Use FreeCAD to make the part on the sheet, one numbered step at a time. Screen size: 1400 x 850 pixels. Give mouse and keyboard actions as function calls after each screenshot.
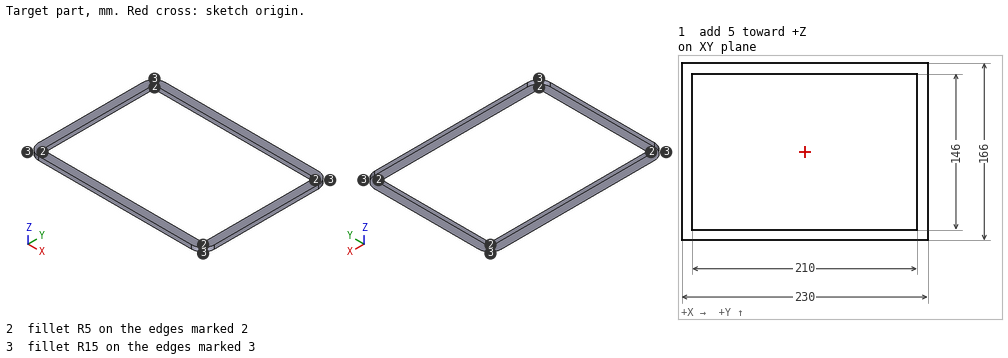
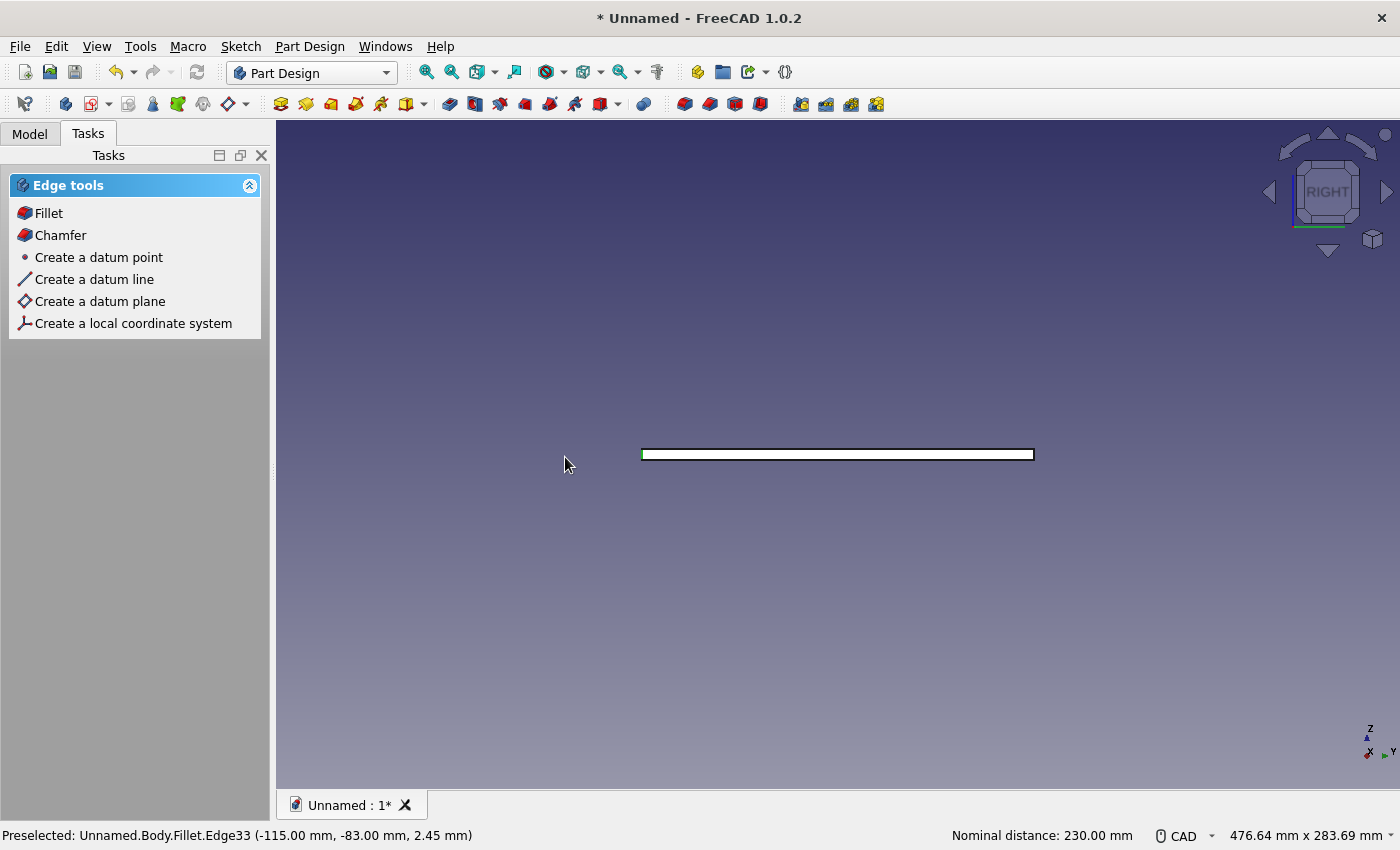
scroll(1034, 453, up, 7)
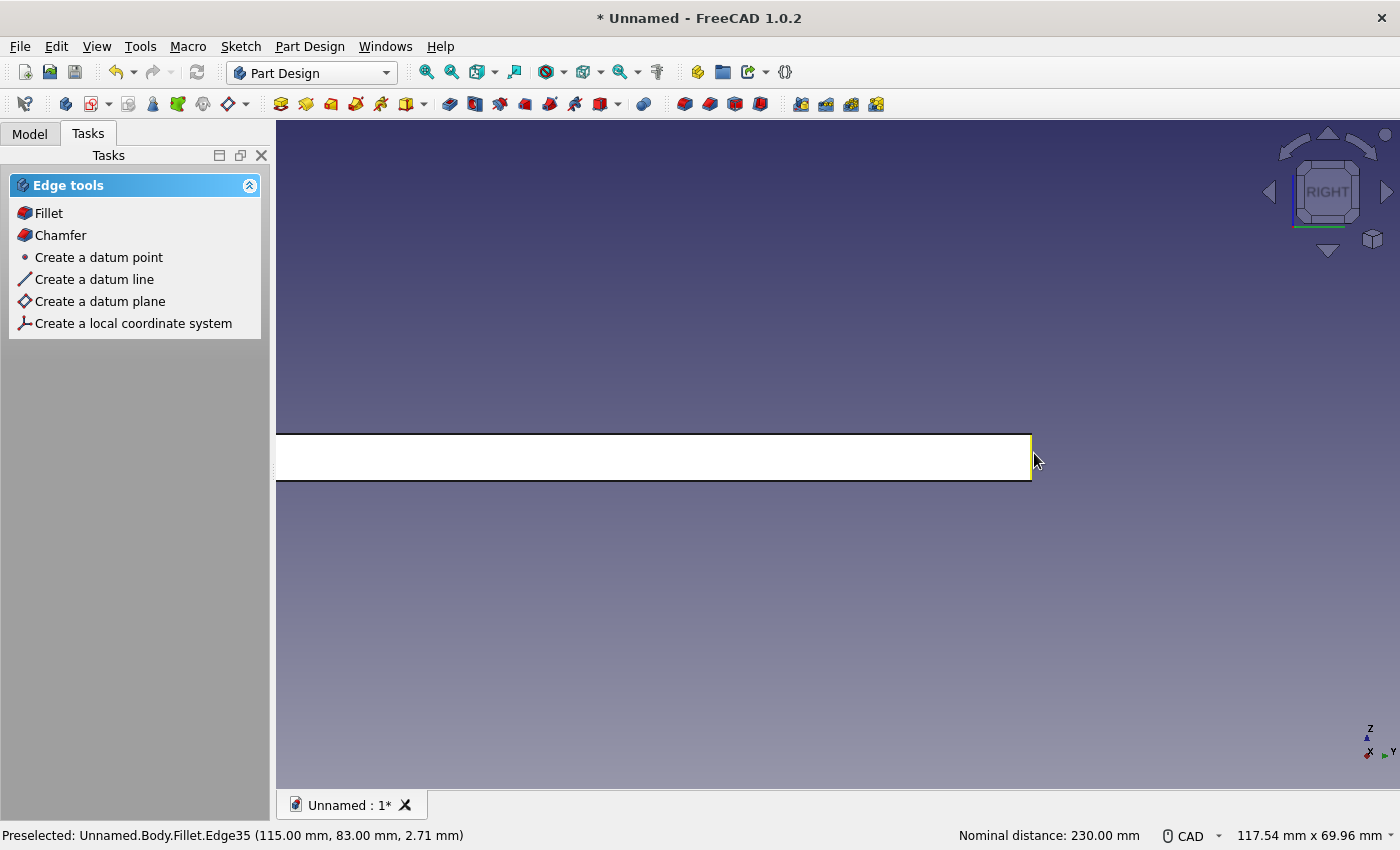
click(1031, 457, ctrl)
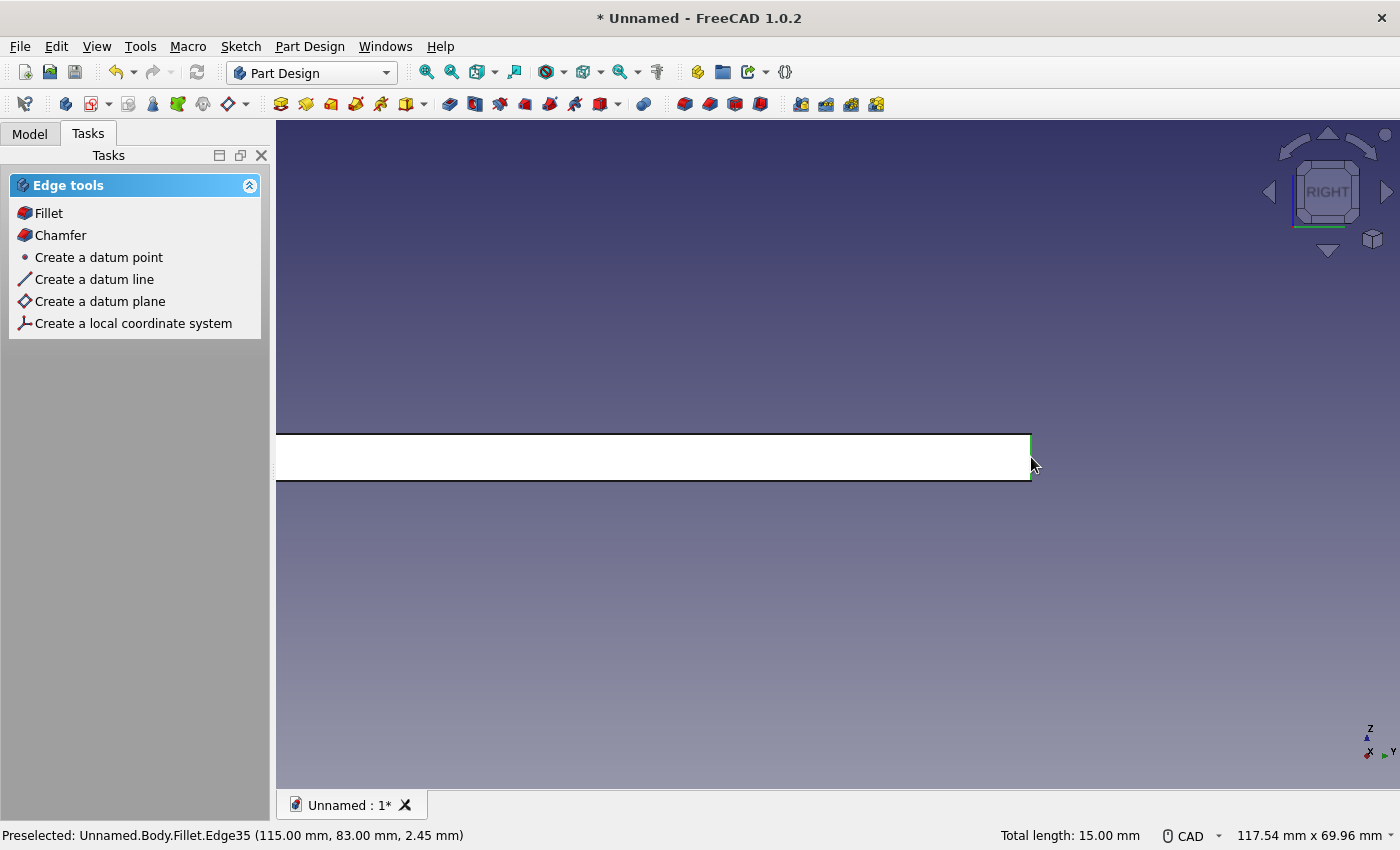
key(v)
key(f)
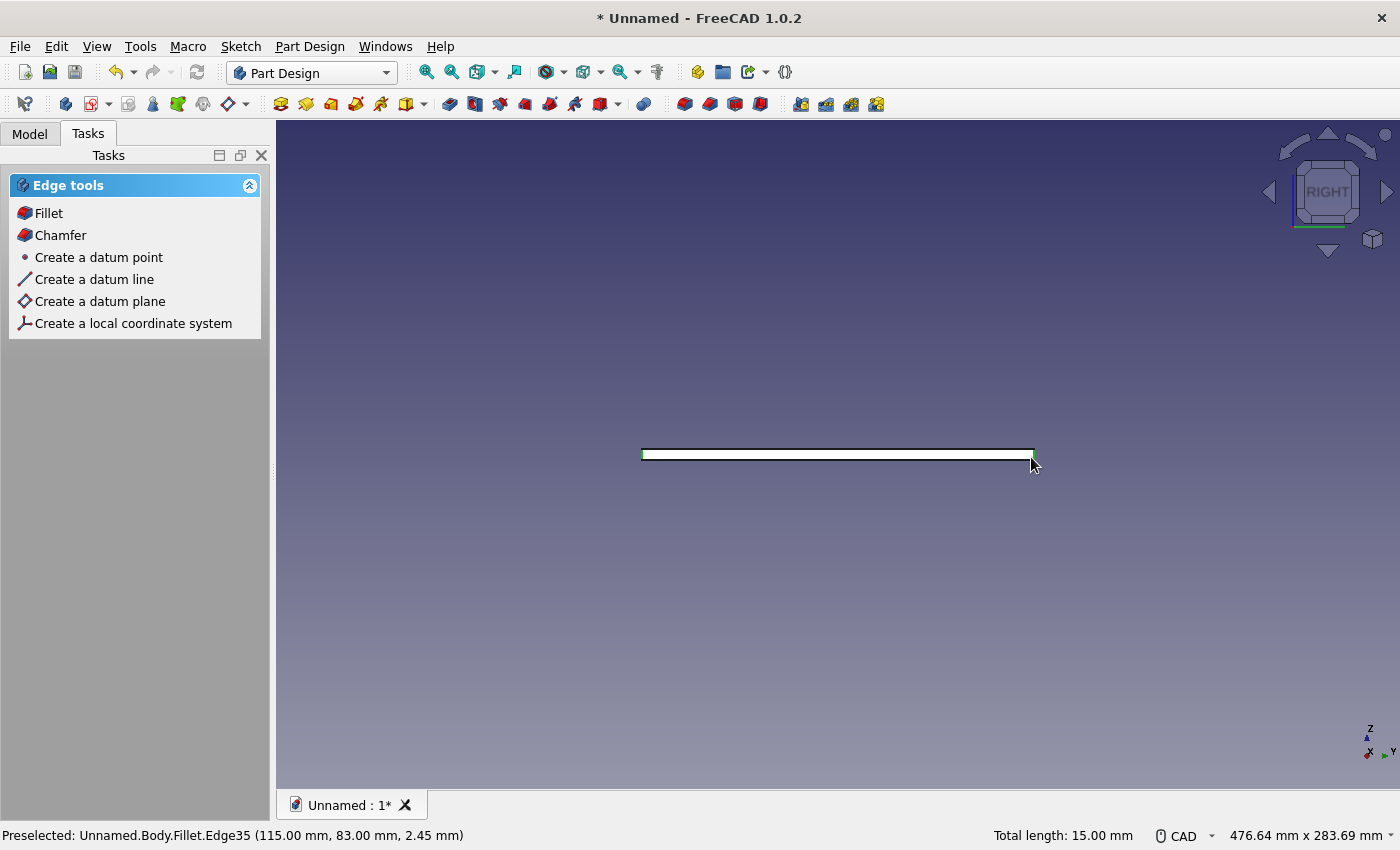
key(5)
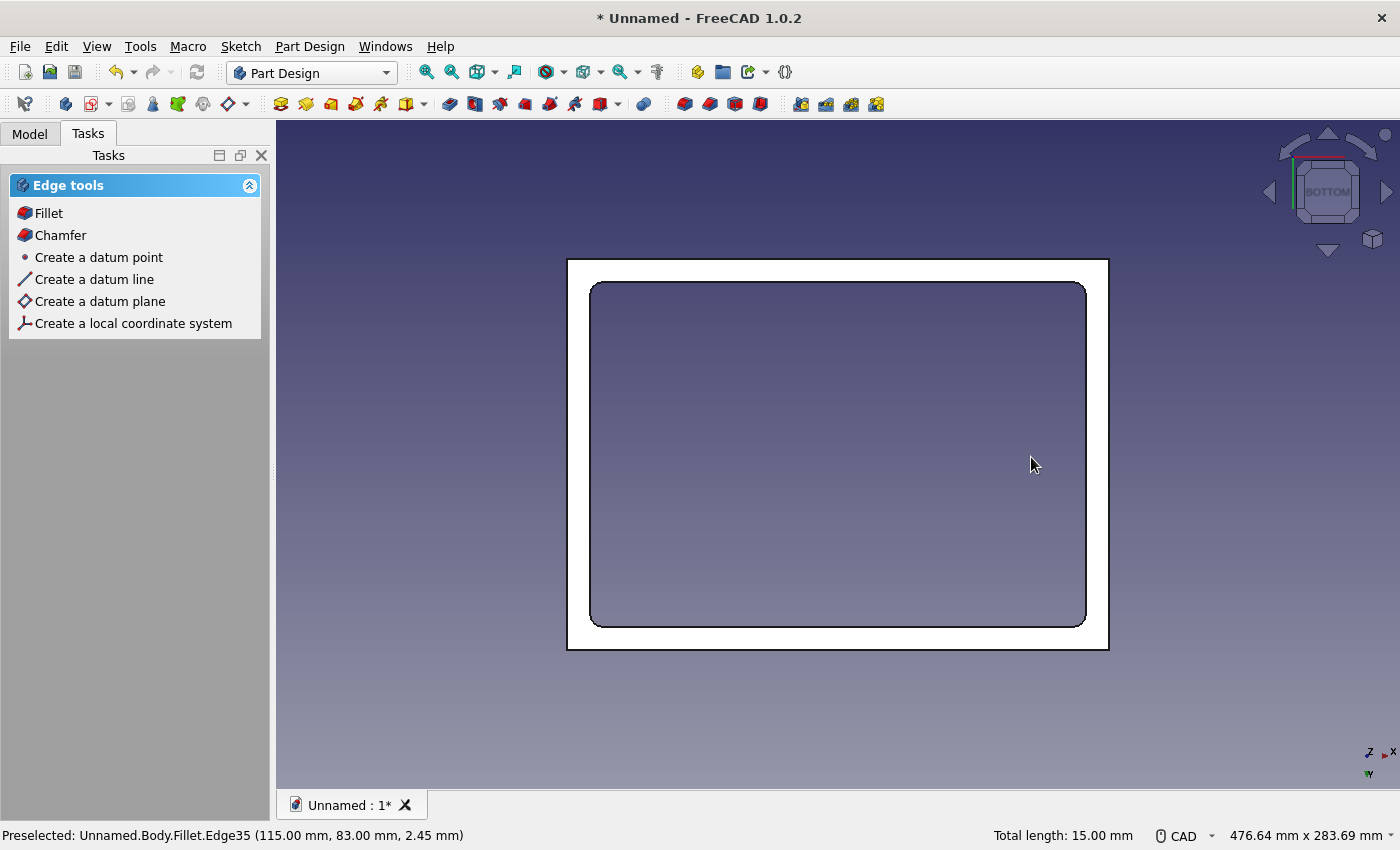
scroll(567, 649, up, 7)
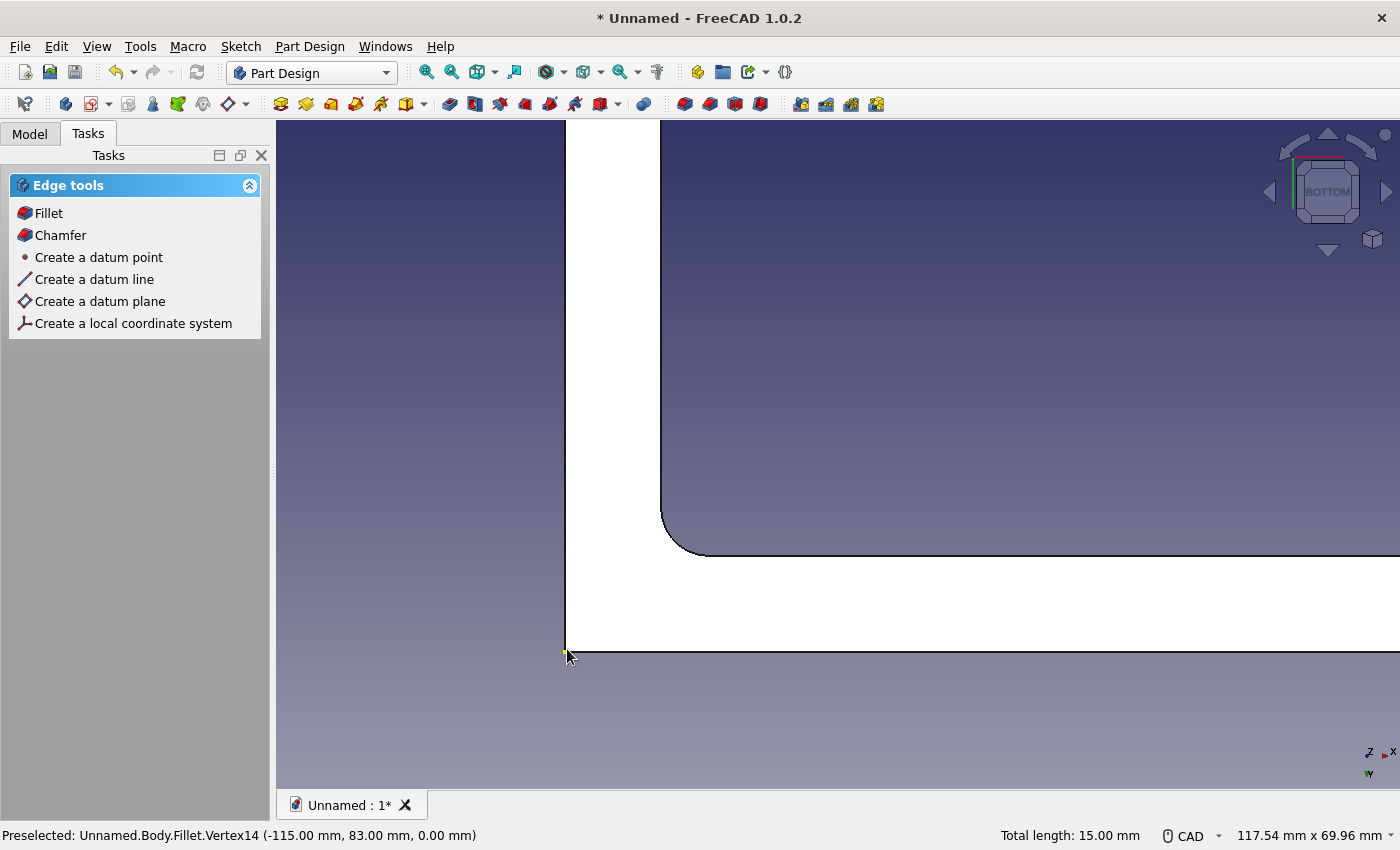
key(v)
key(f)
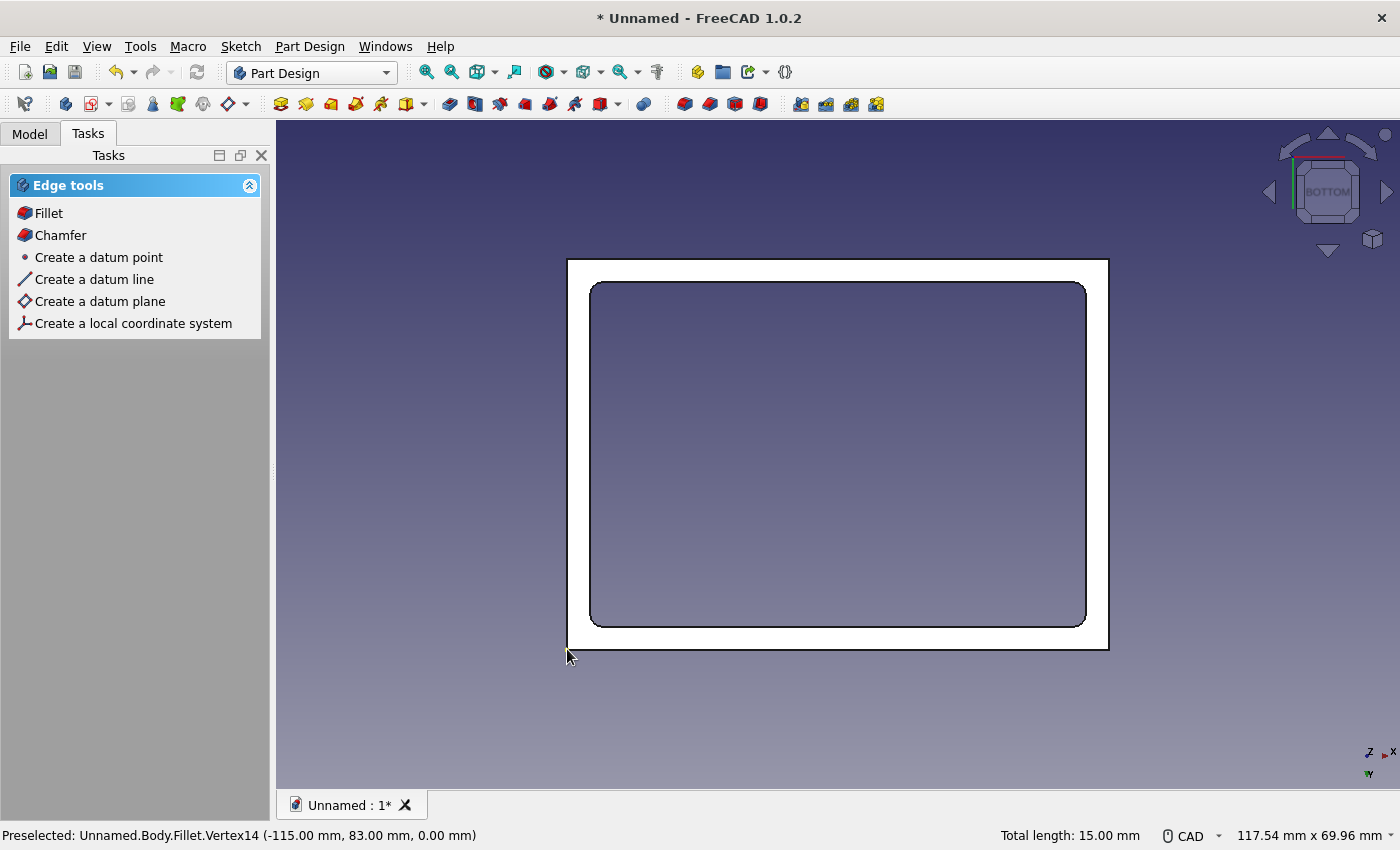
key(4)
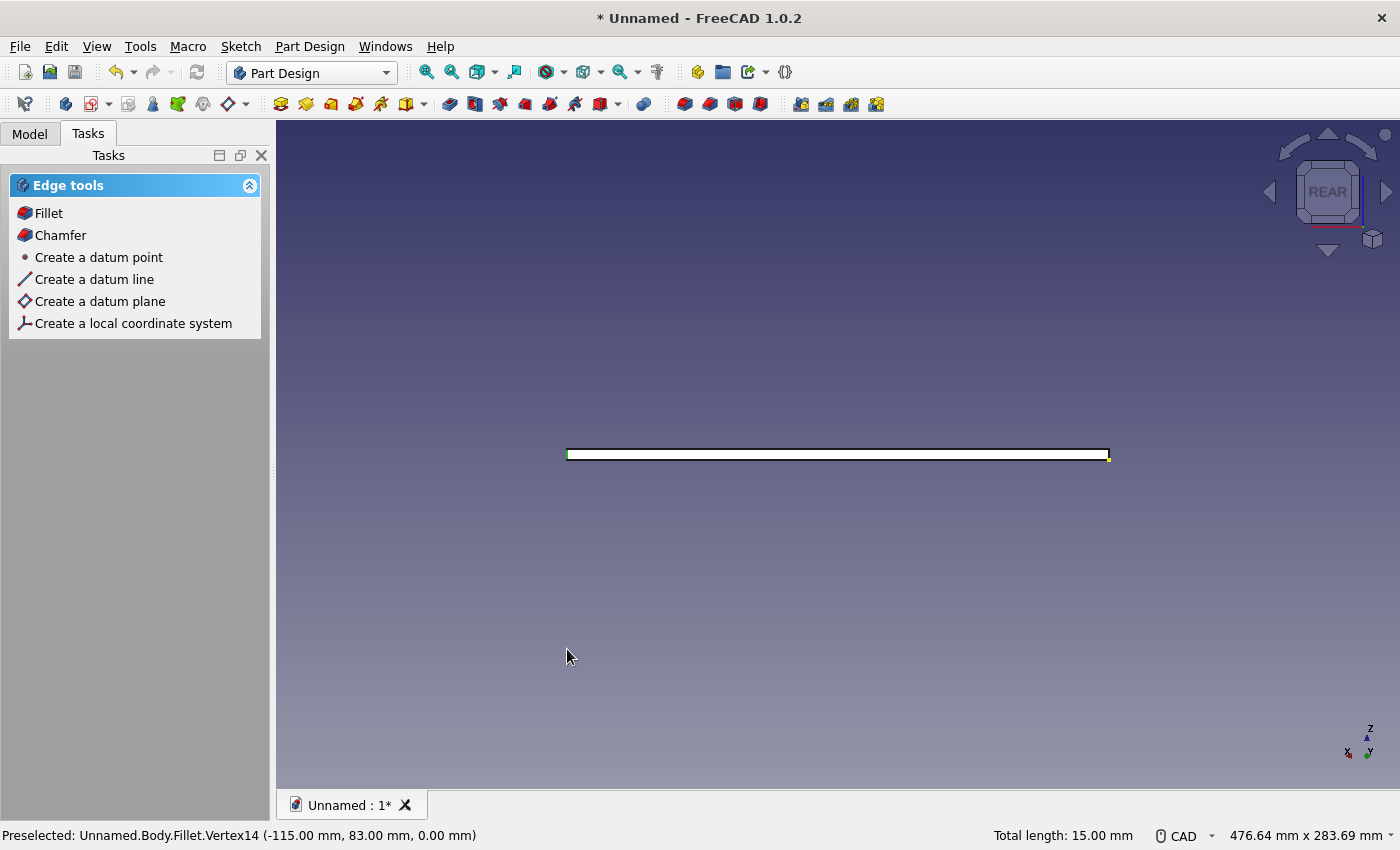
scroll(1109, 453, up, 7)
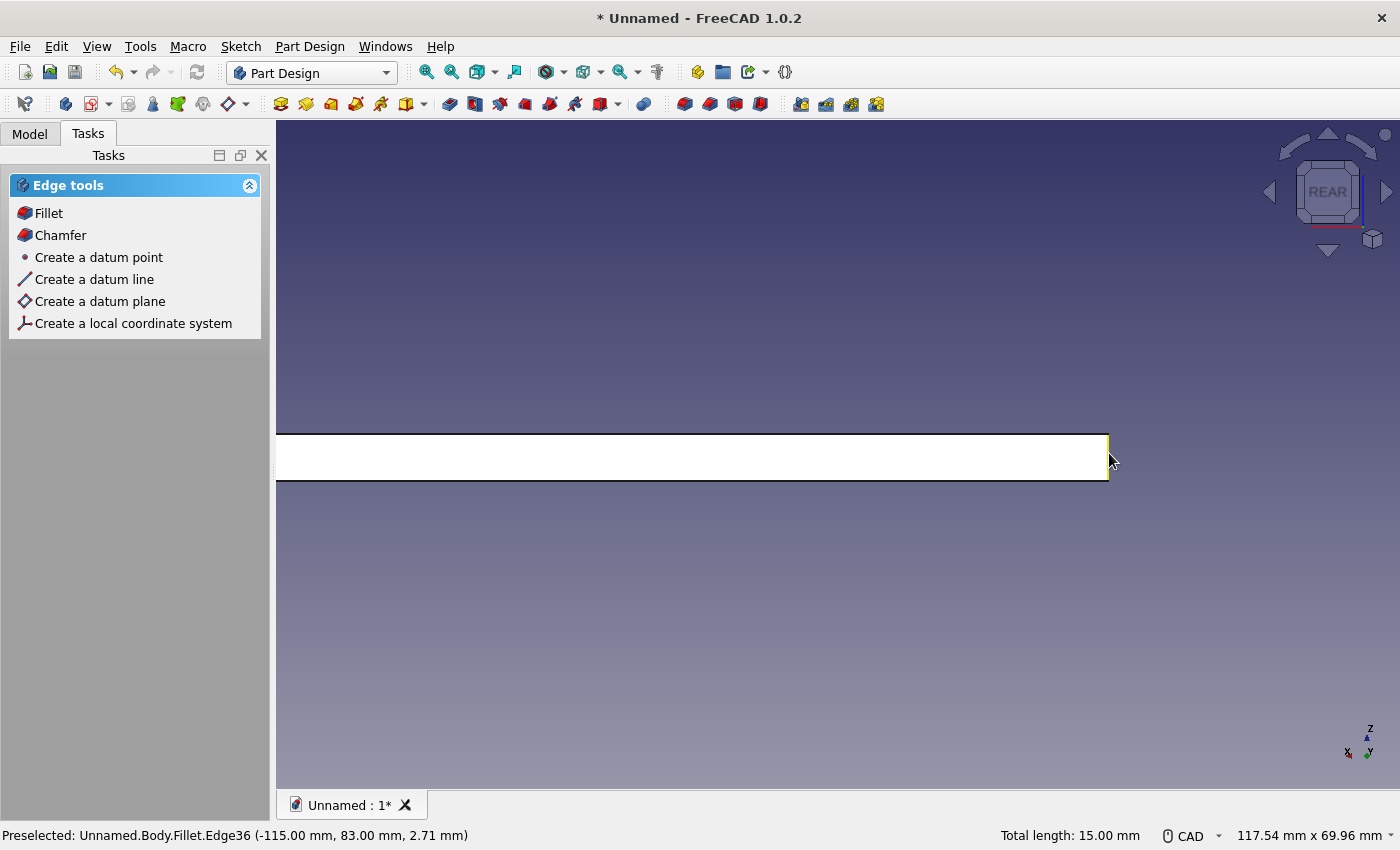
click(1108, 457, ctrl)